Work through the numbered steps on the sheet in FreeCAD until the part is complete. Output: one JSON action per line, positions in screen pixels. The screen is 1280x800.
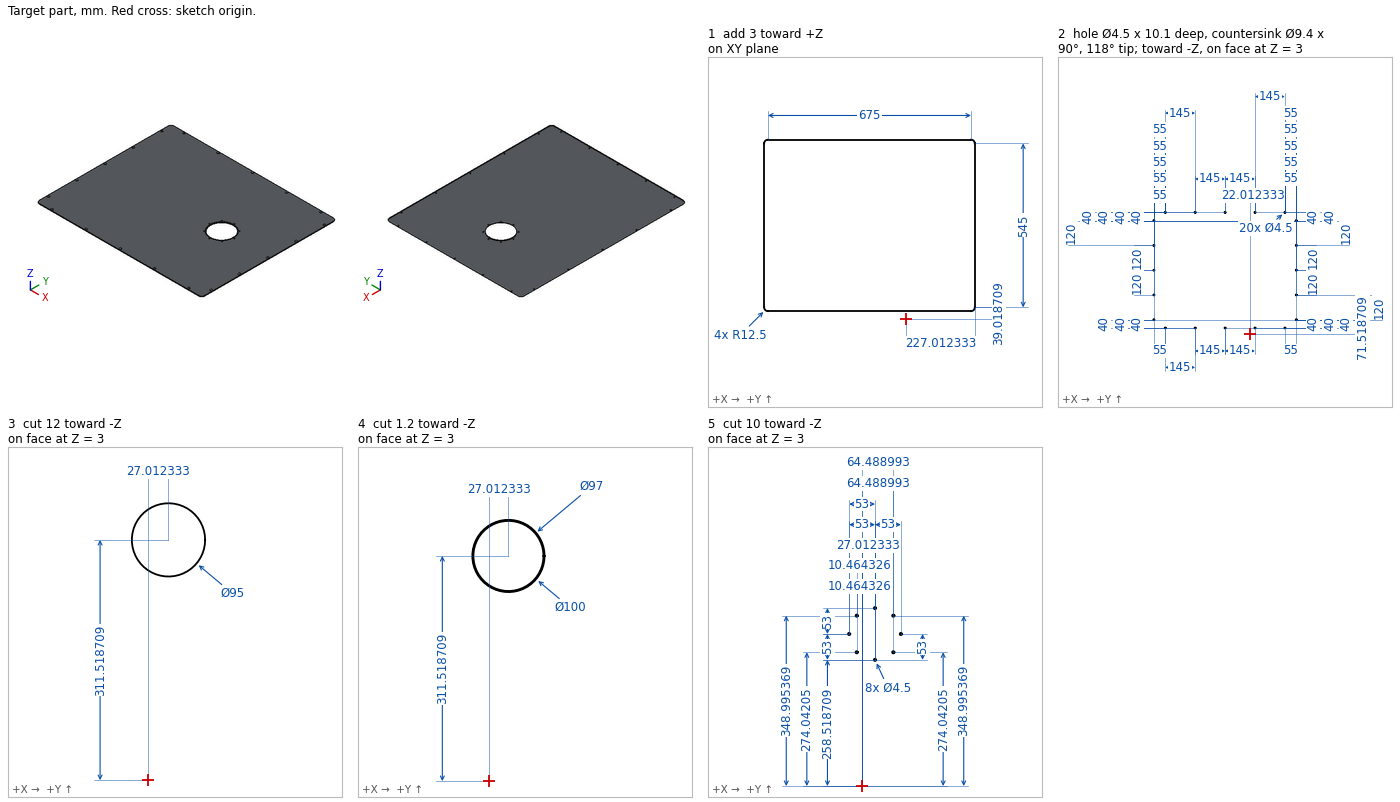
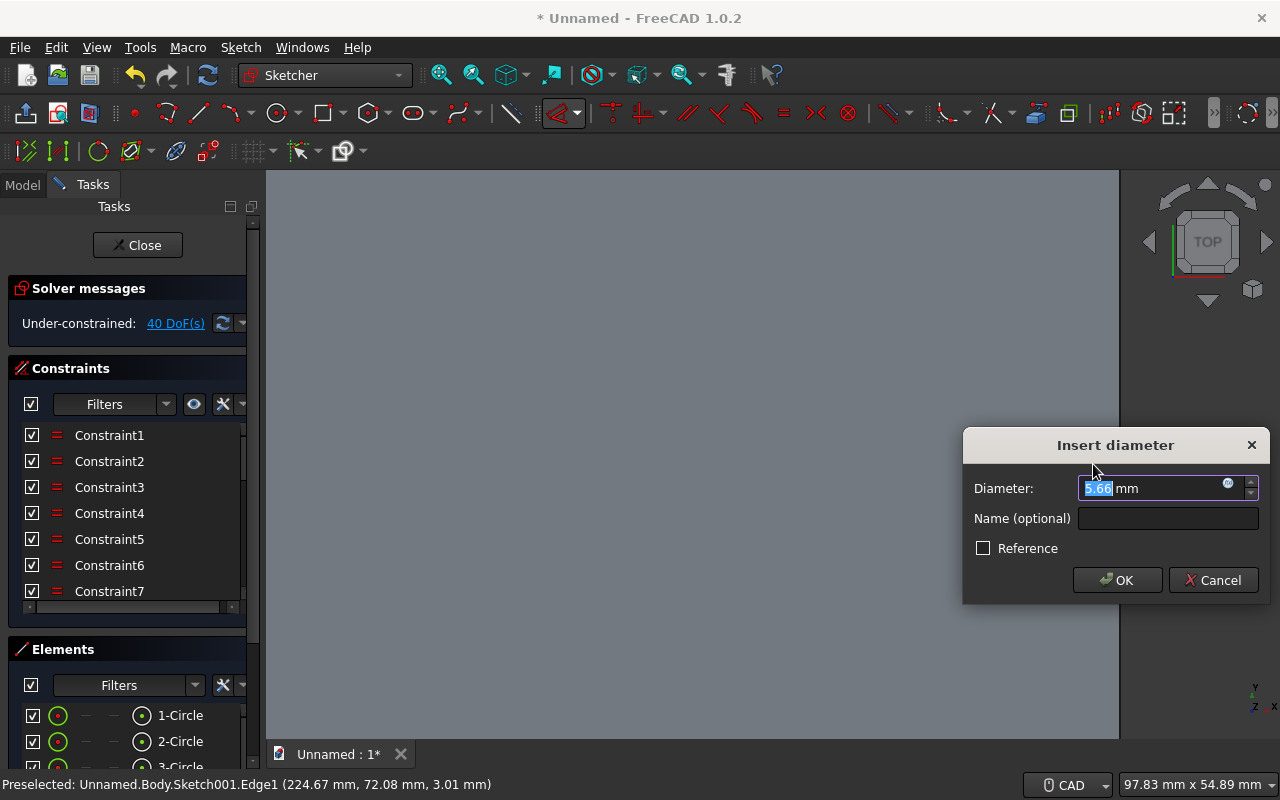
{"action": "type", "text": "4.5"}
{"action": "key", "text": "Return"}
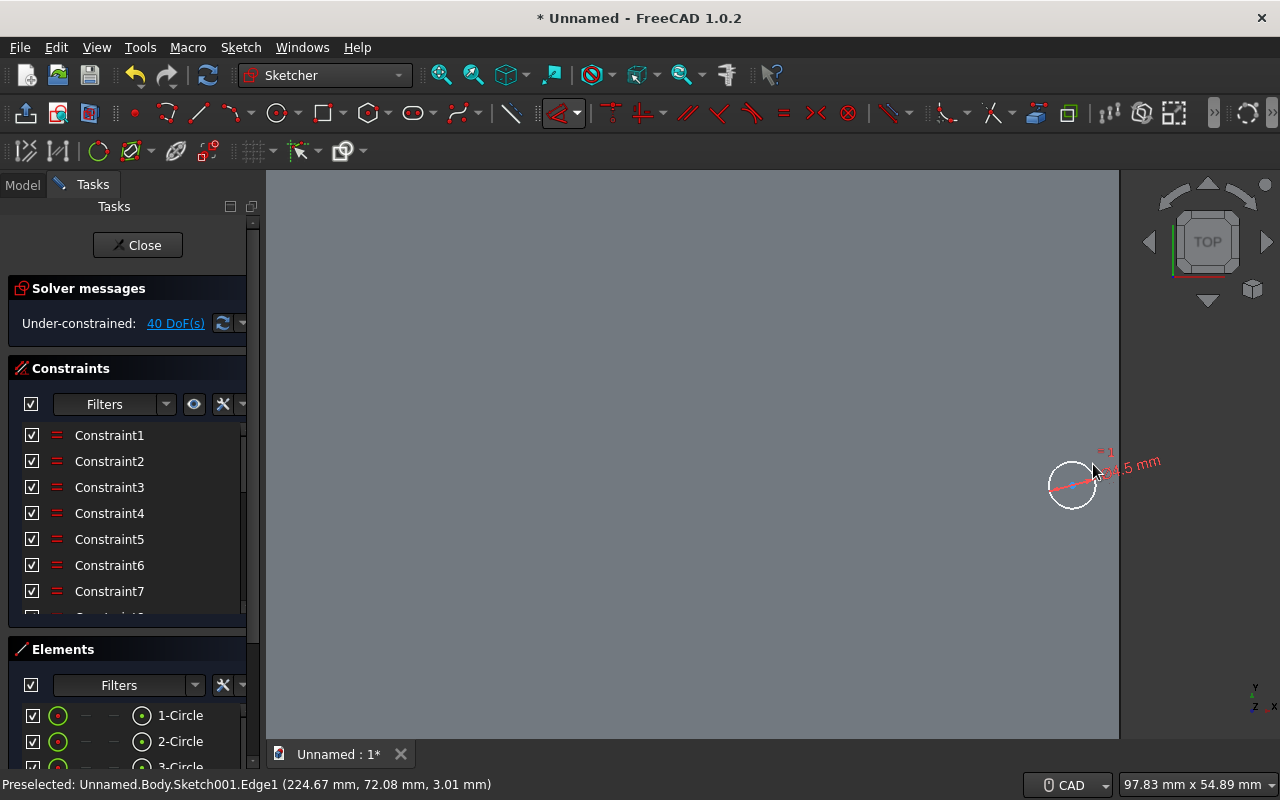
{"action": "scroll", "coordinate": [912, 604], "scroll_direction": "down", "scroll_amount": 14}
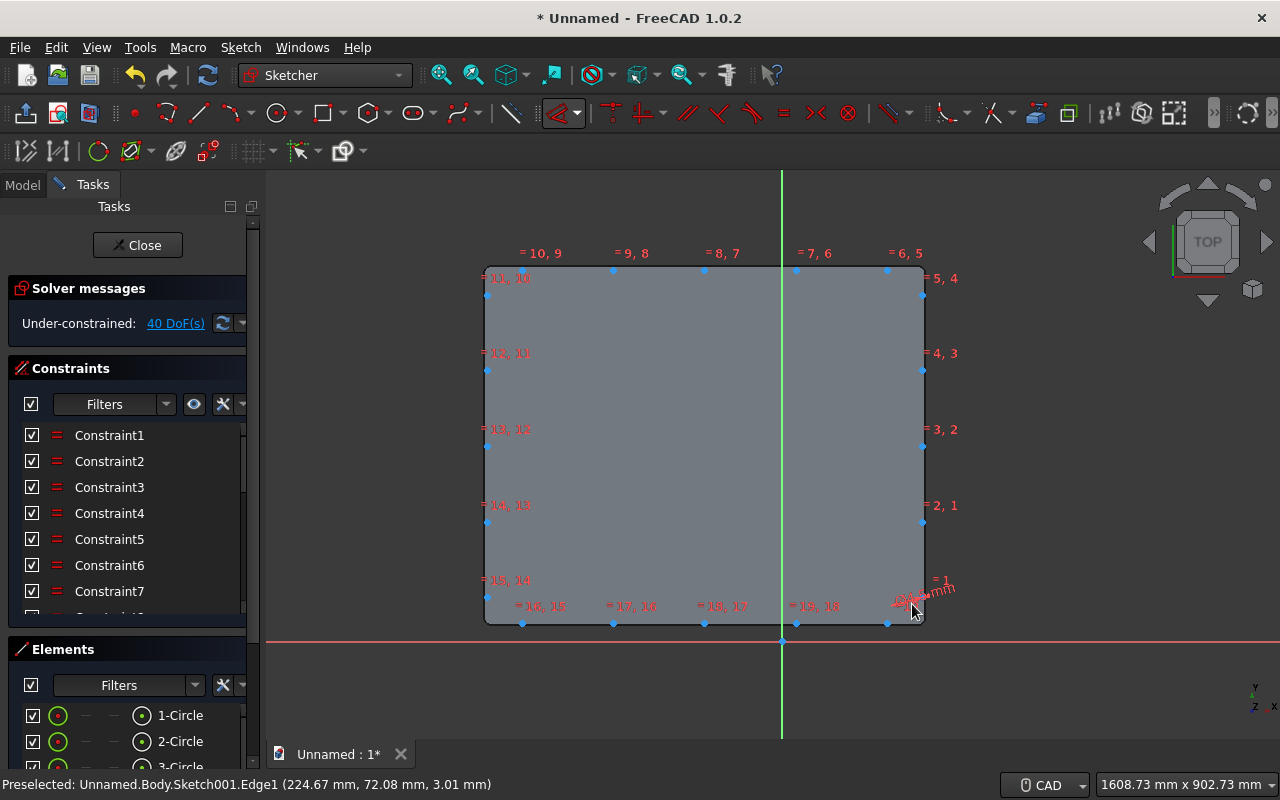
{"action": "left_click", "coordinate": [922, 295]}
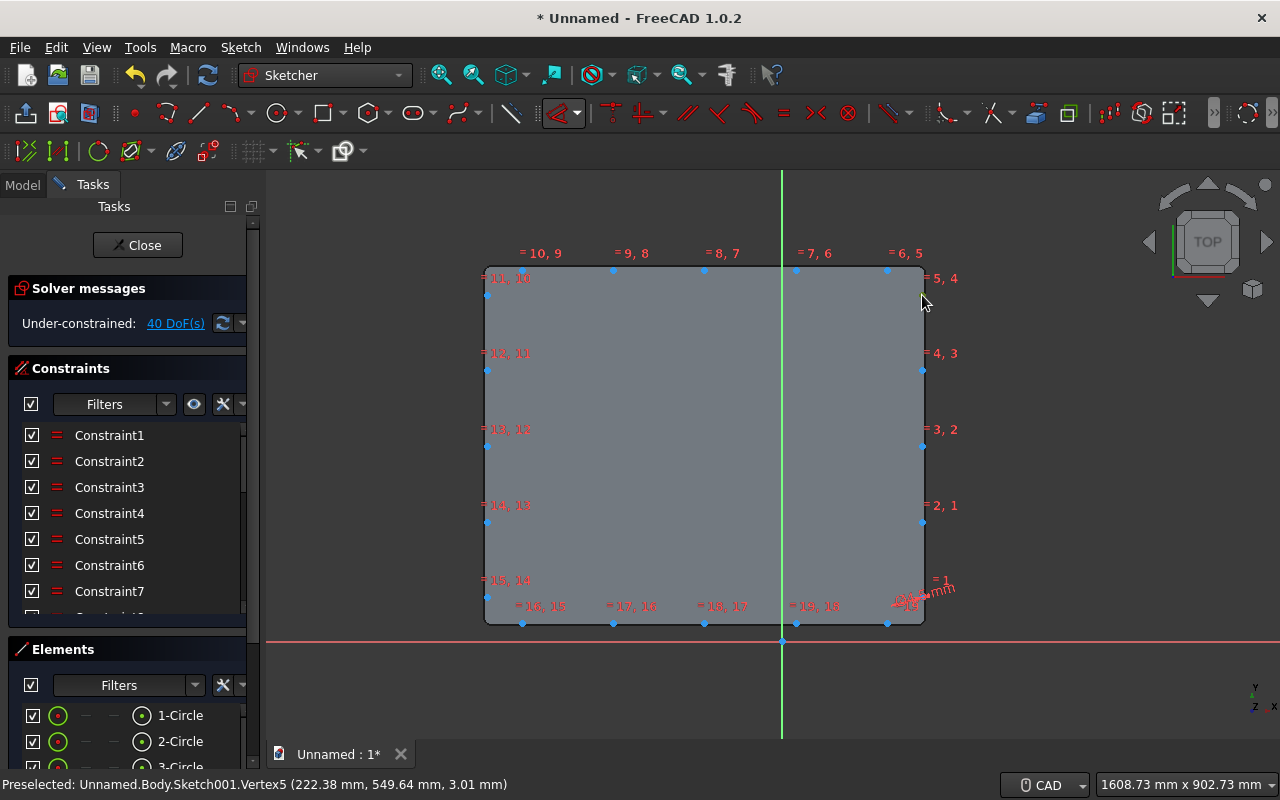
{"action": "left_click", "coordinate": [887, 270]}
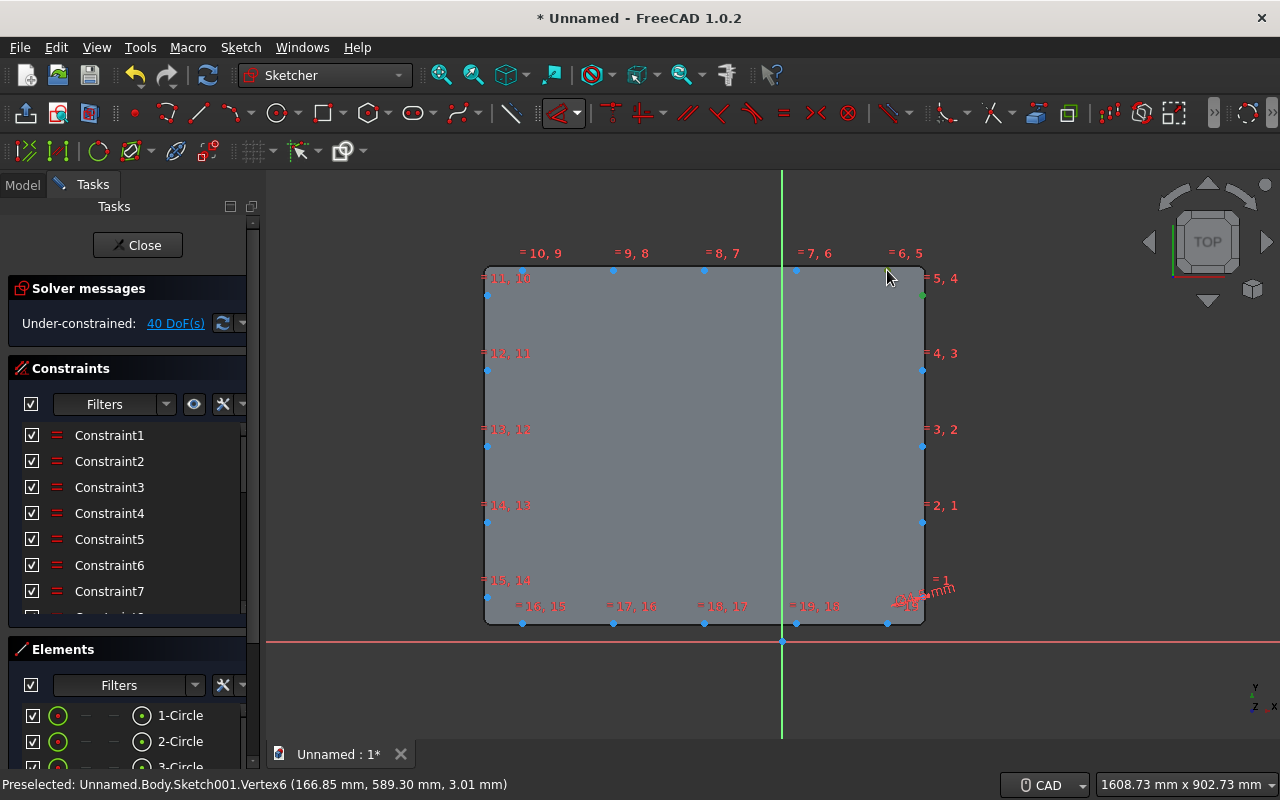
{"action": "left_click", "coordinate": [580, 114]}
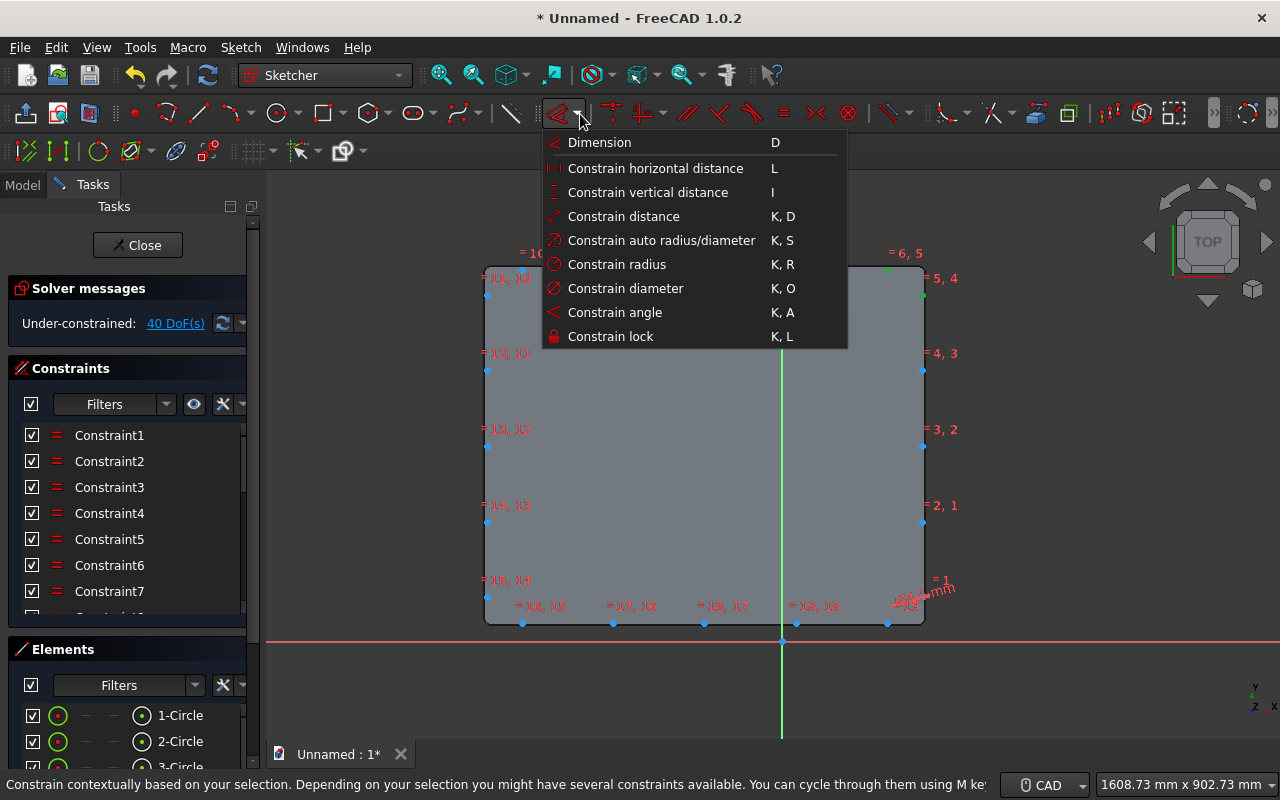
{"action": "left_click", "coordinate": [695, 168]}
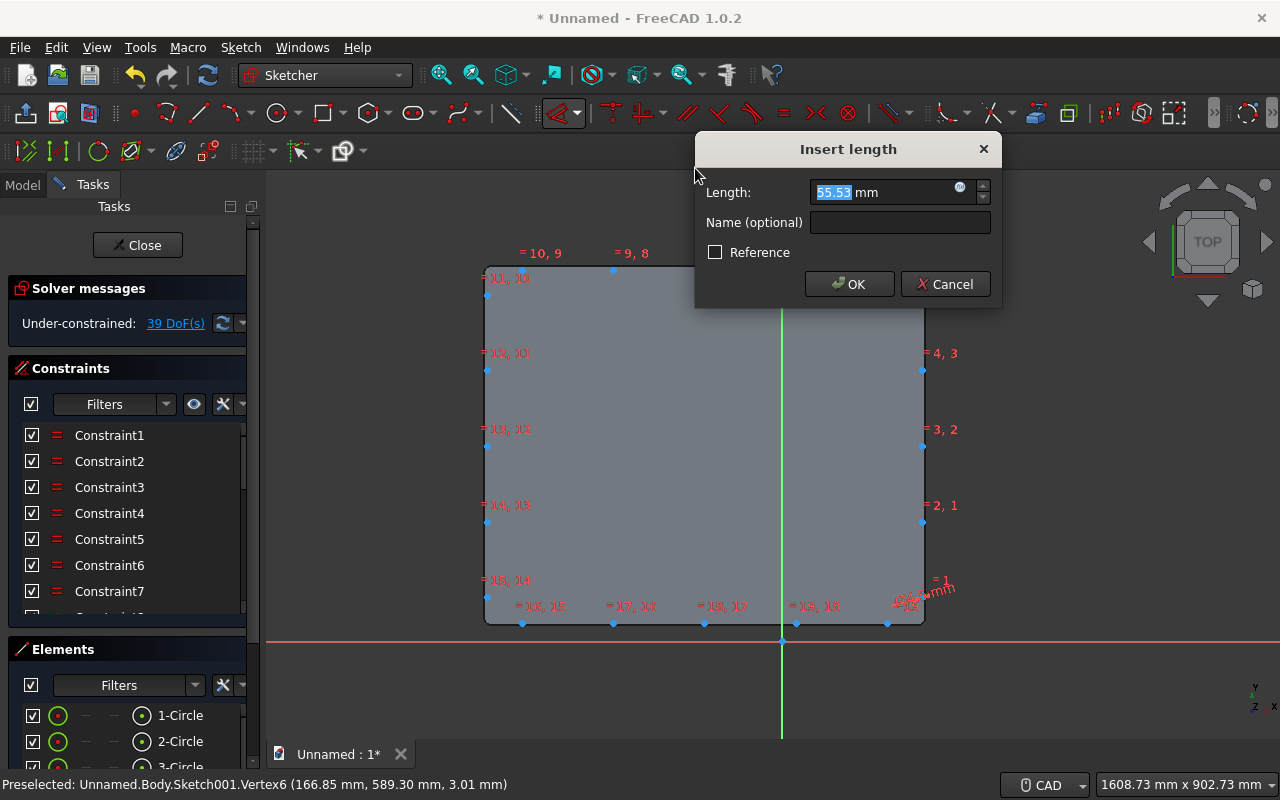
{"action": "type", "text": "55"}
{"action": "key", "text": "Return"}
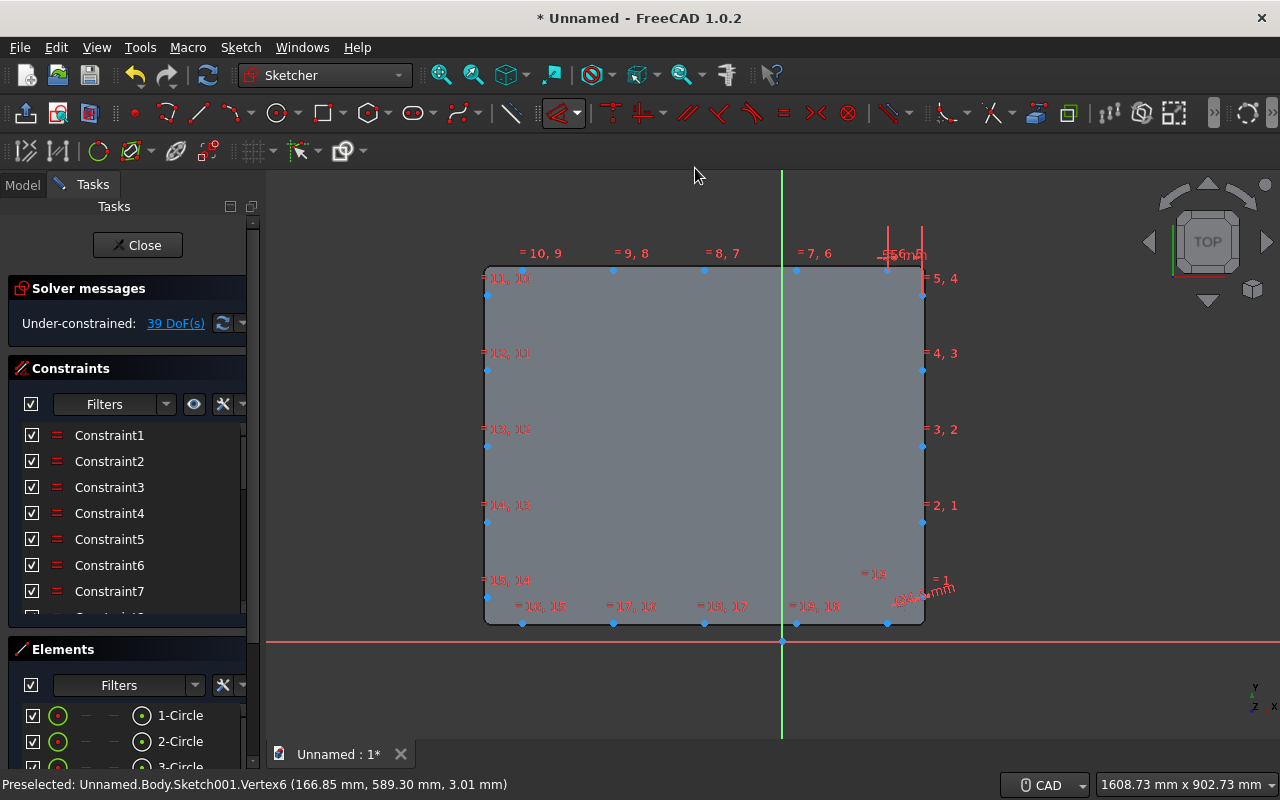
{"action": "left_click", "coordinate": [922, 370]}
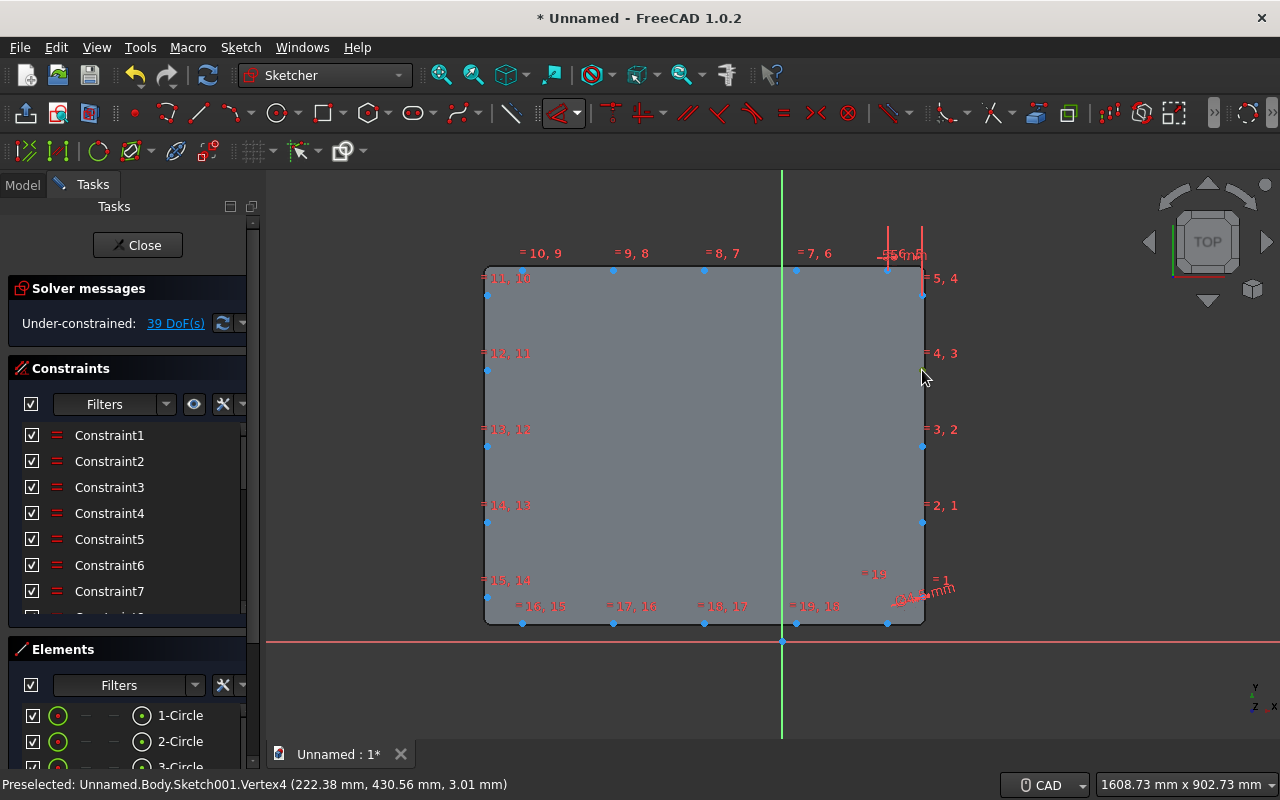
{"action": "left_click", "coordinate": [888, 270]}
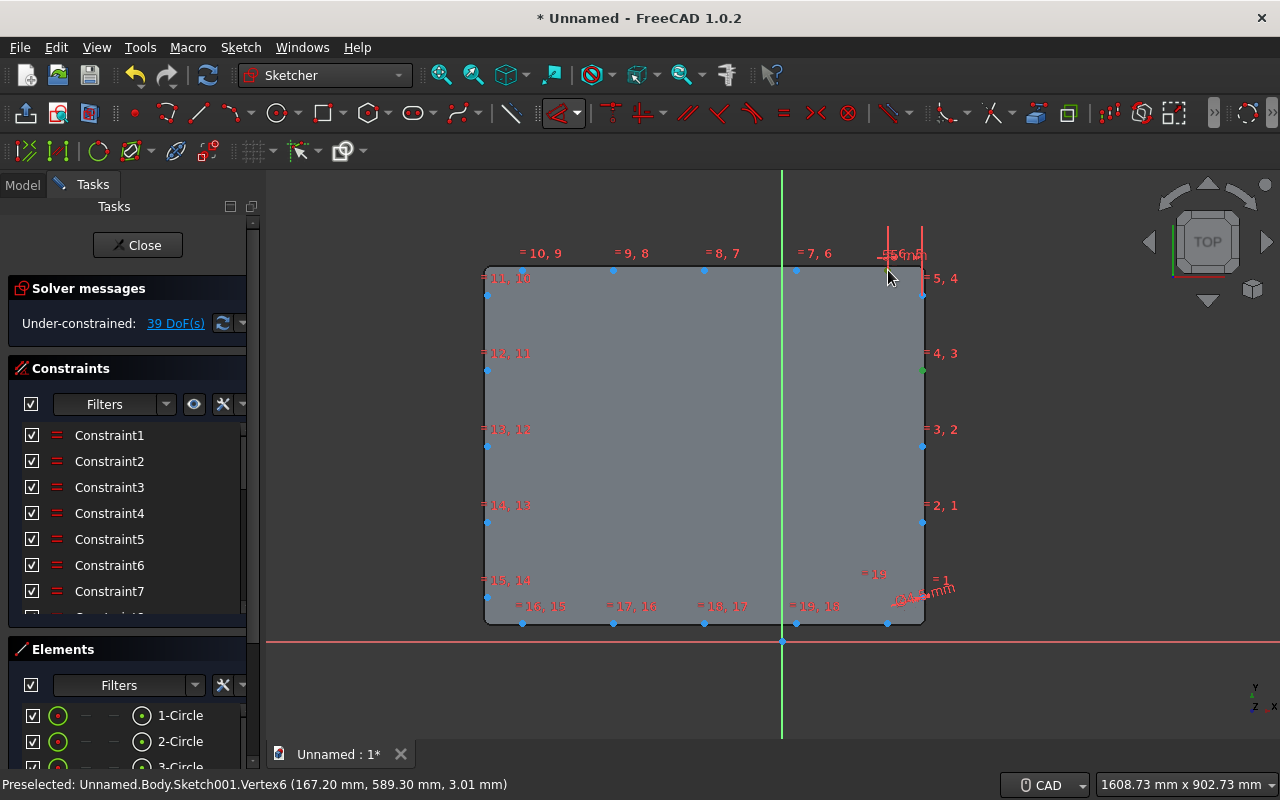
{"action": "key", "text": "l"}